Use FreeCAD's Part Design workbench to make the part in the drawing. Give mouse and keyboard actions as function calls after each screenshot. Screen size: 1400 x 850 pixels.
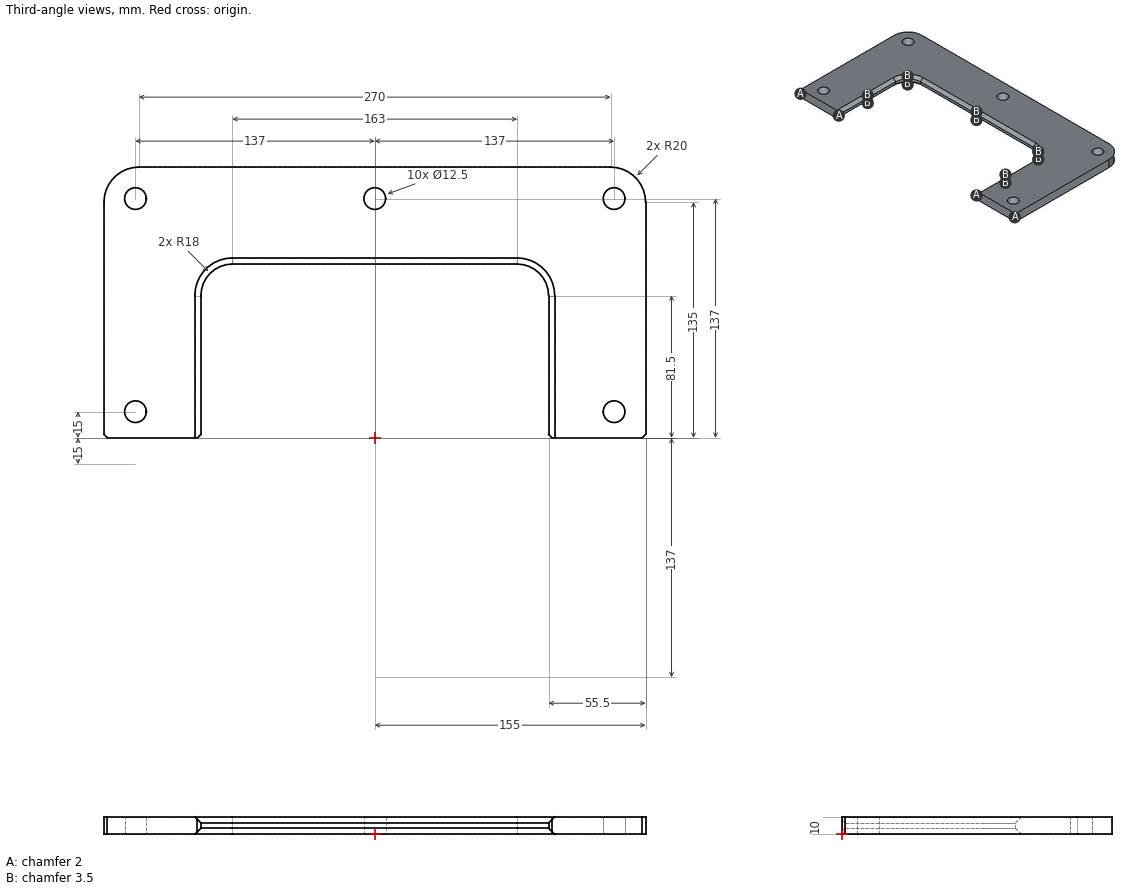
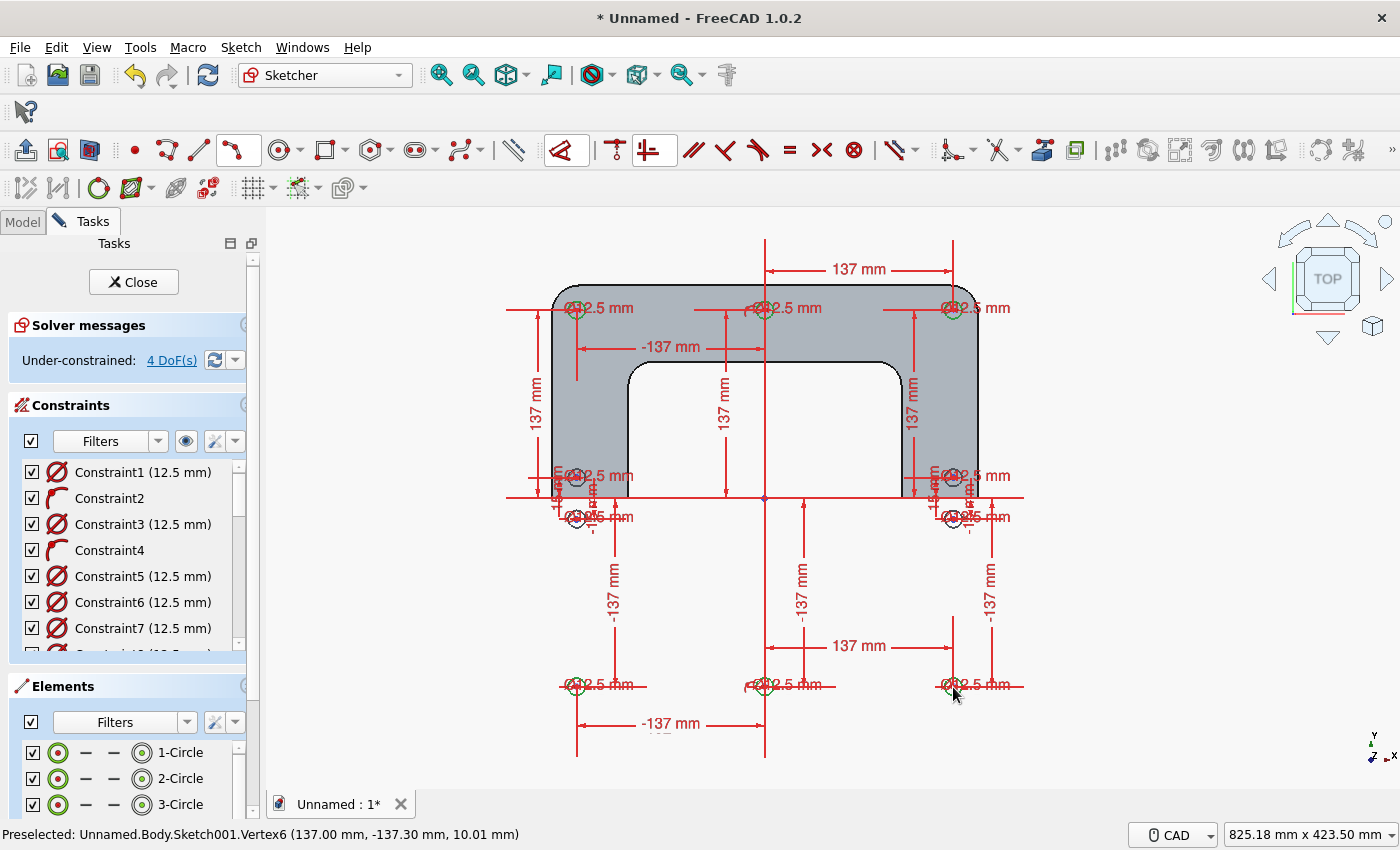
click(577, 478)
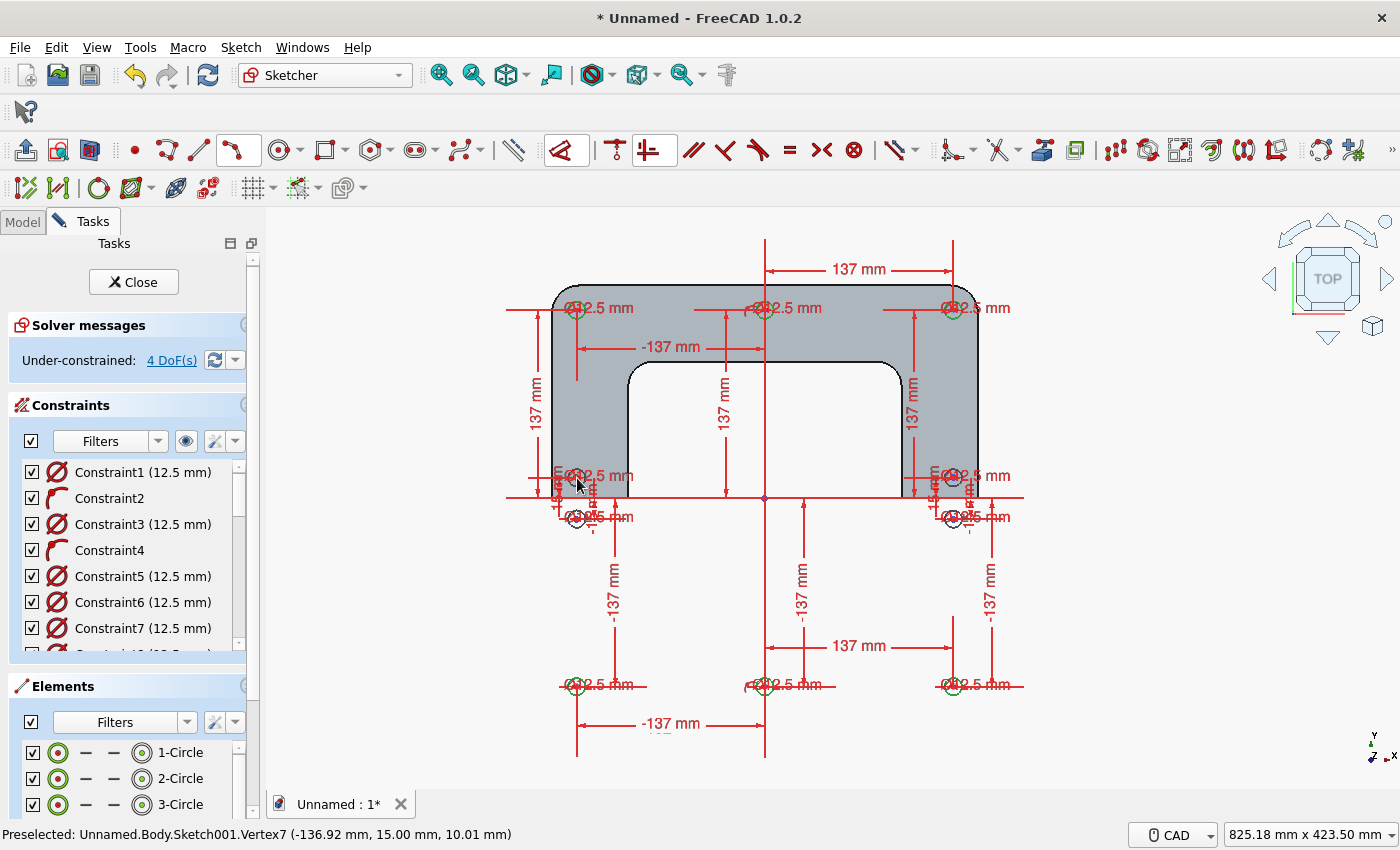
key(l)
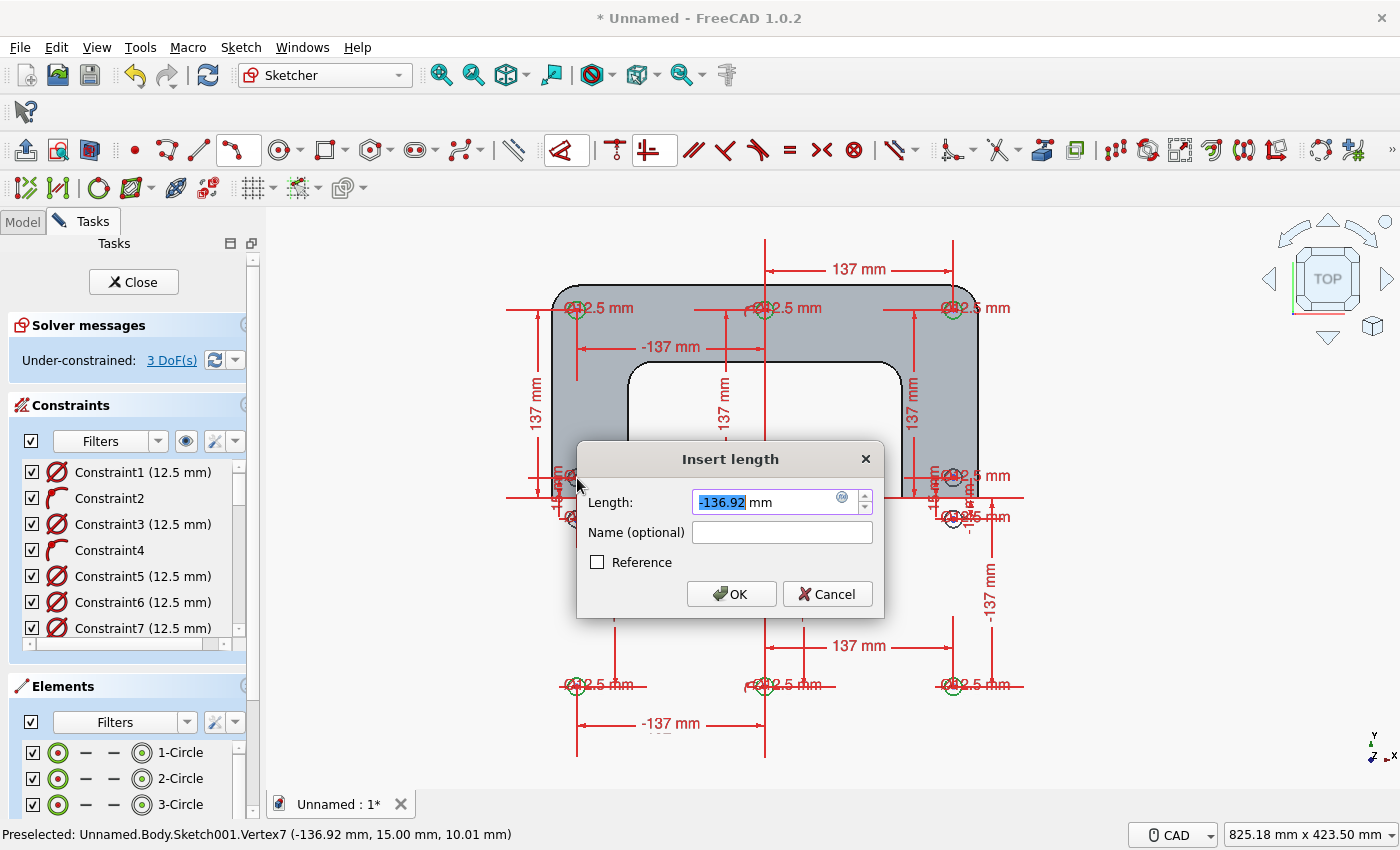
text(-137)
key(Return)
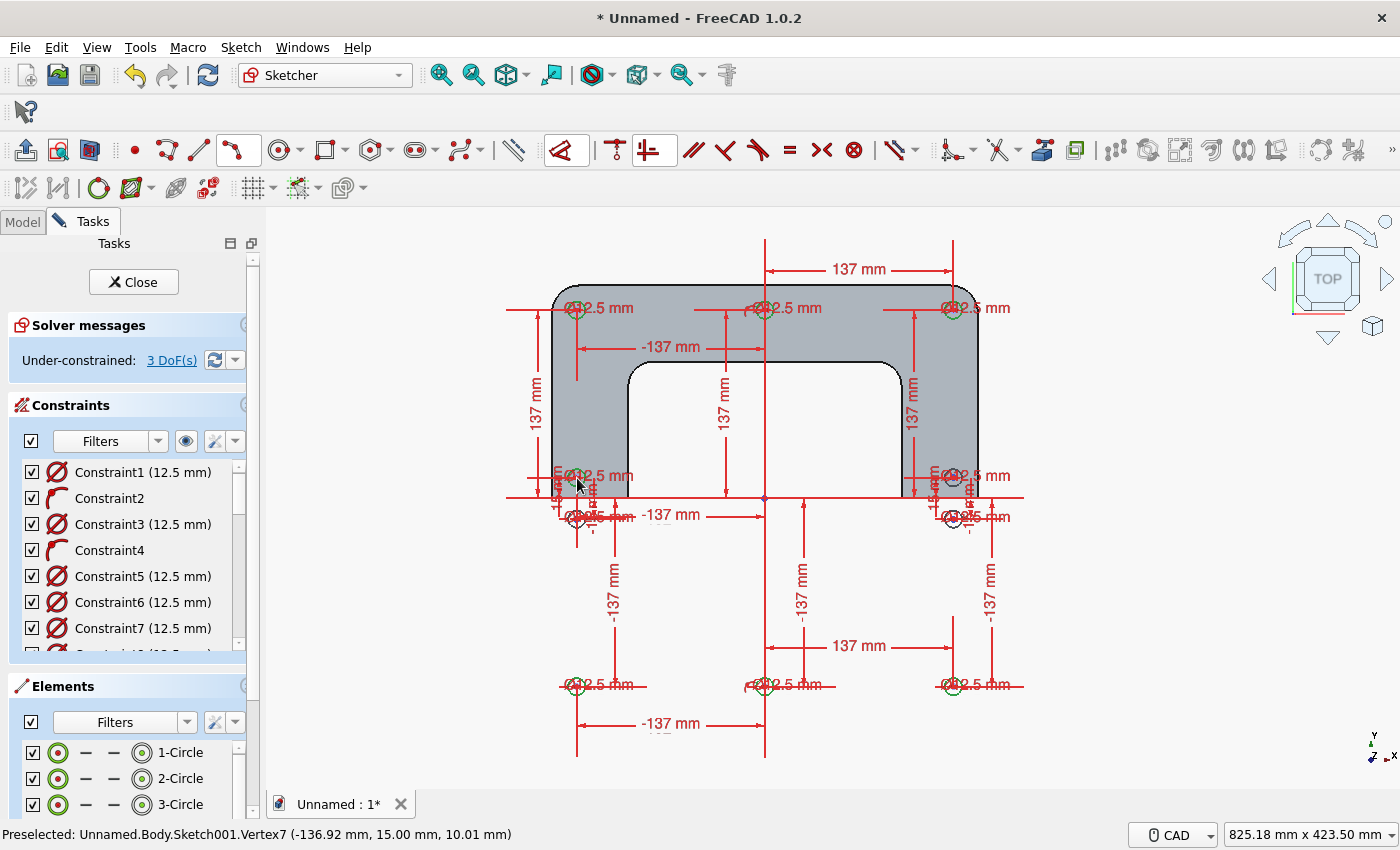
click(577, 519)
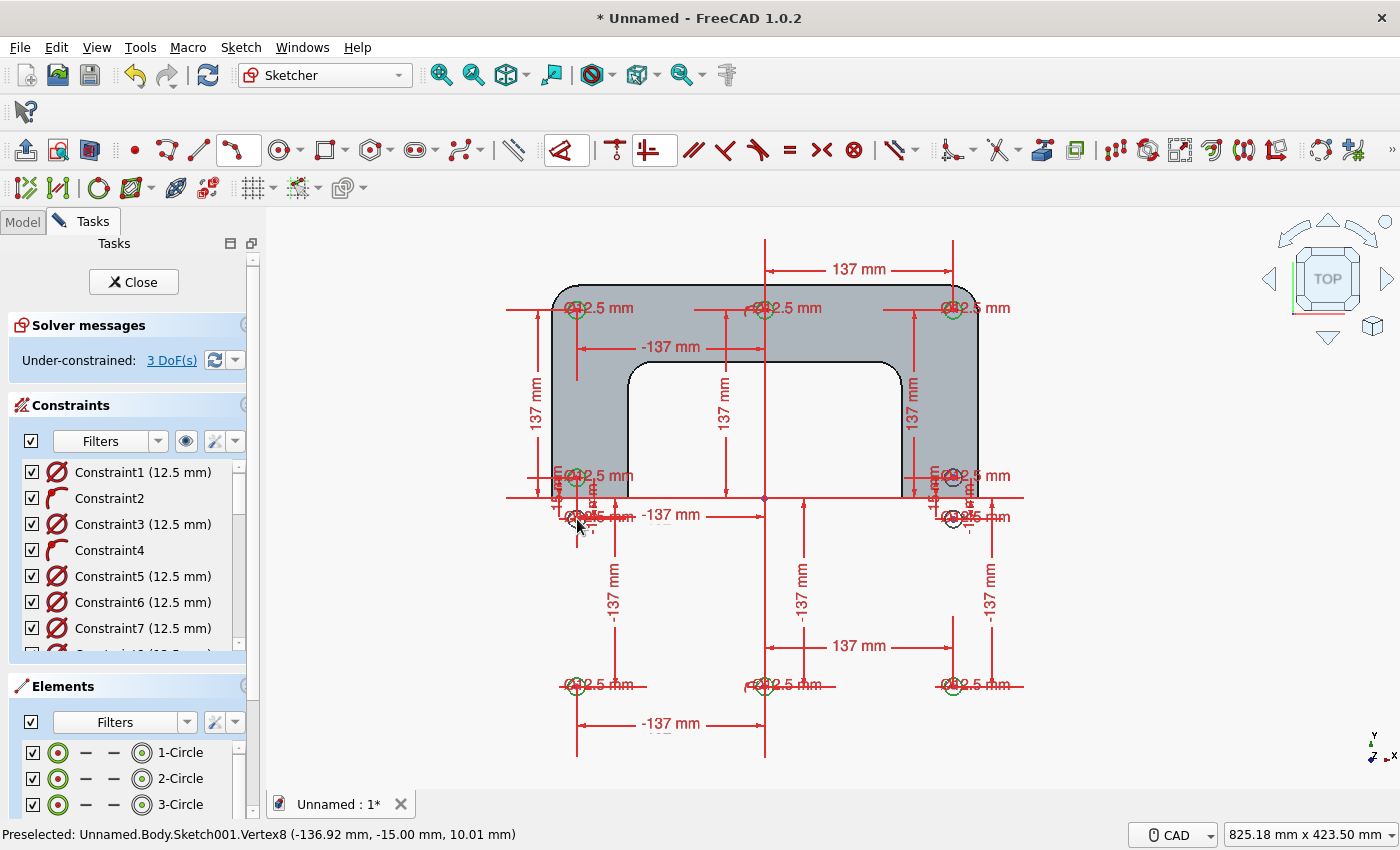
click(584, 150)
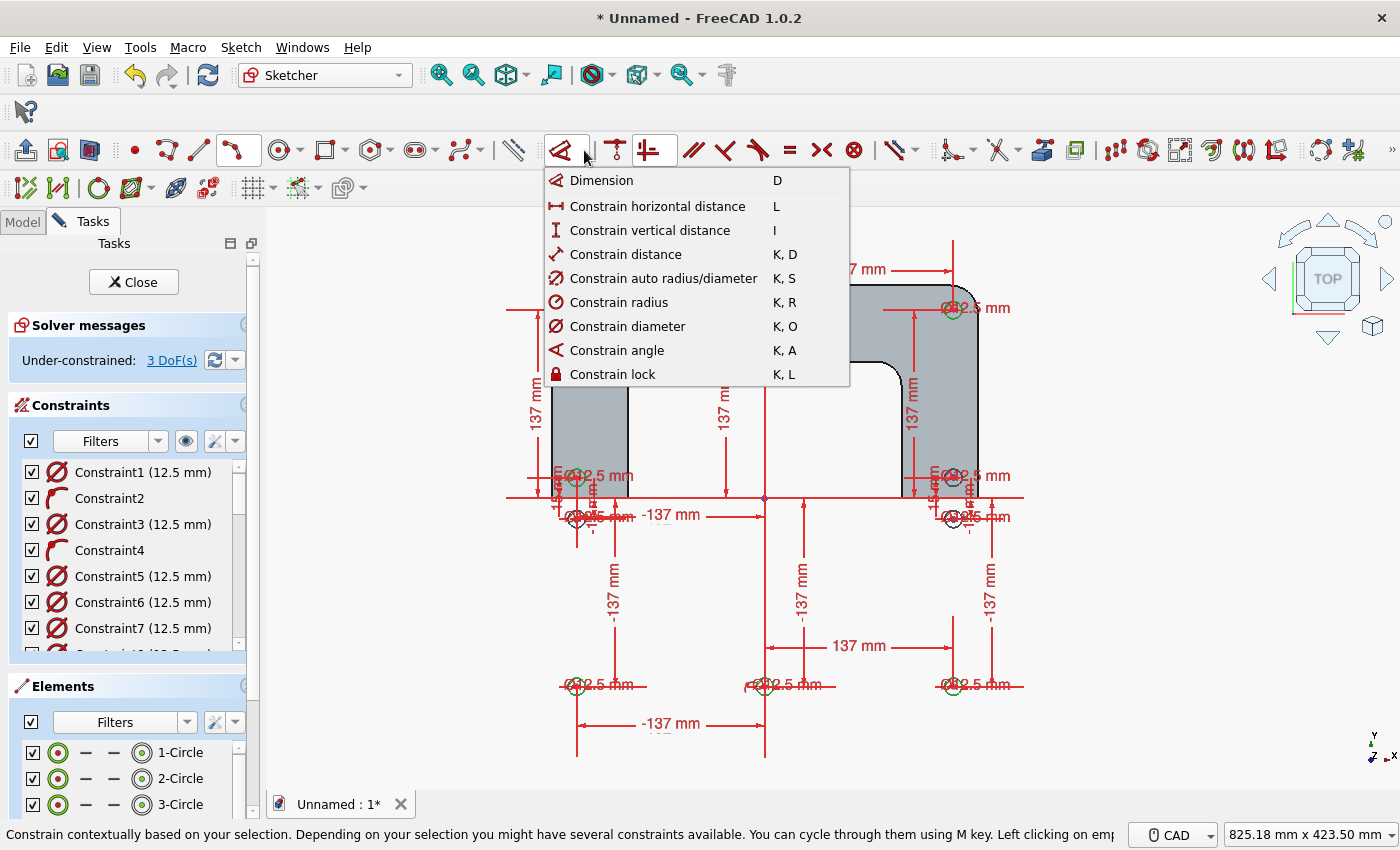
click(697, 206)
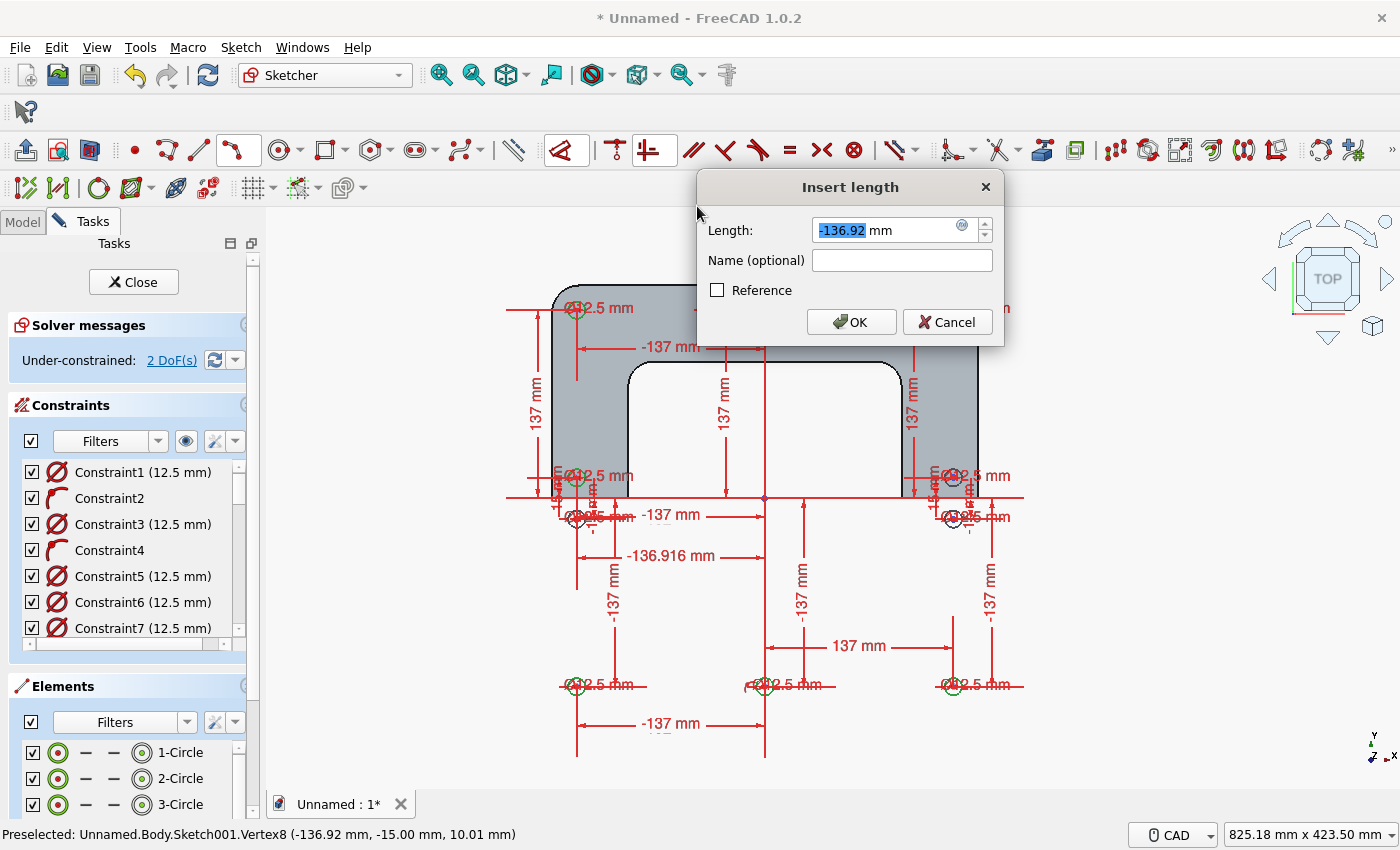
text(-137)
key(Return)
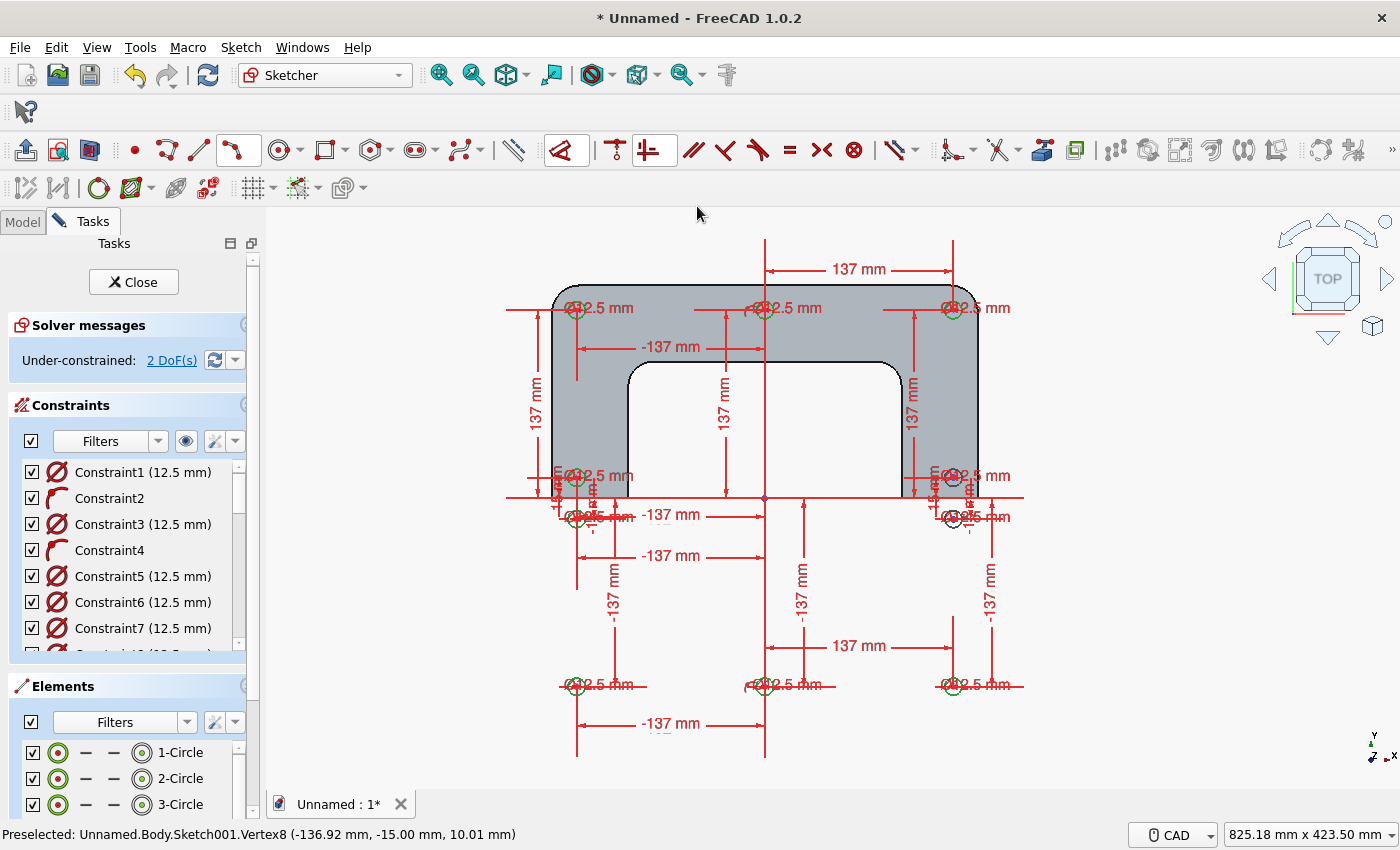
click(953, 519)